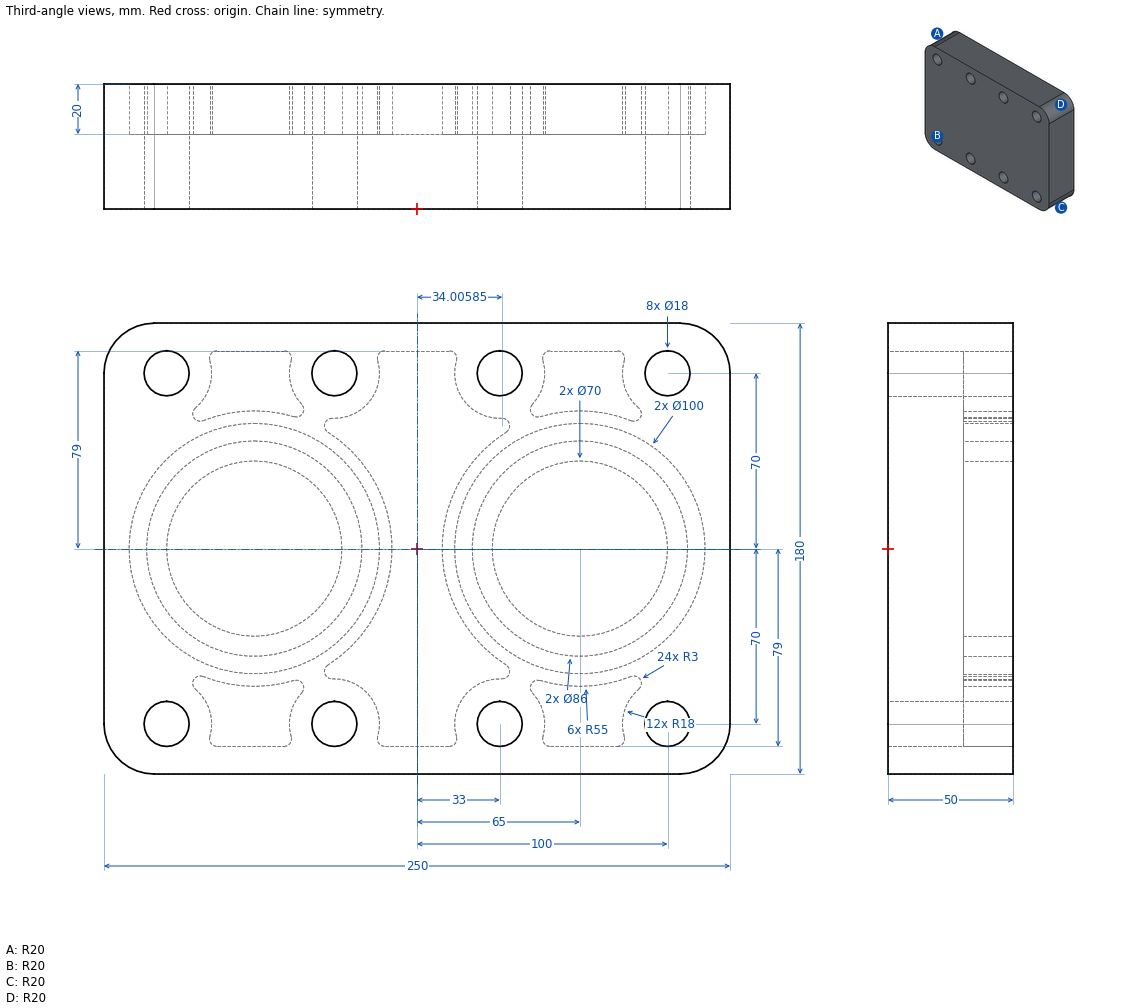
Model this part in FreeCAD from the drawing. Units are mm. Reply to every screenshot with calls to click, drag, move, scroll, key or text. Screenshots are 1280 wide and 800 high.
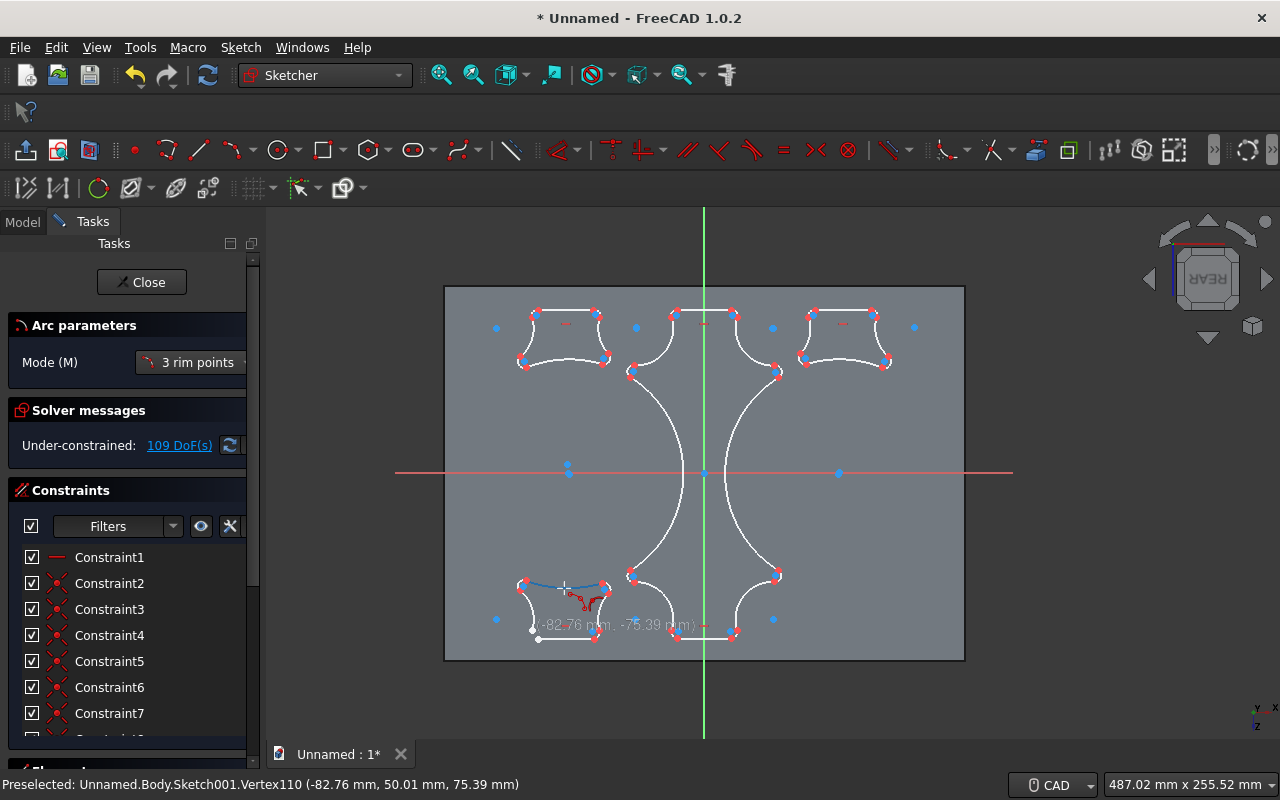
scroll(538, 638, up, 3)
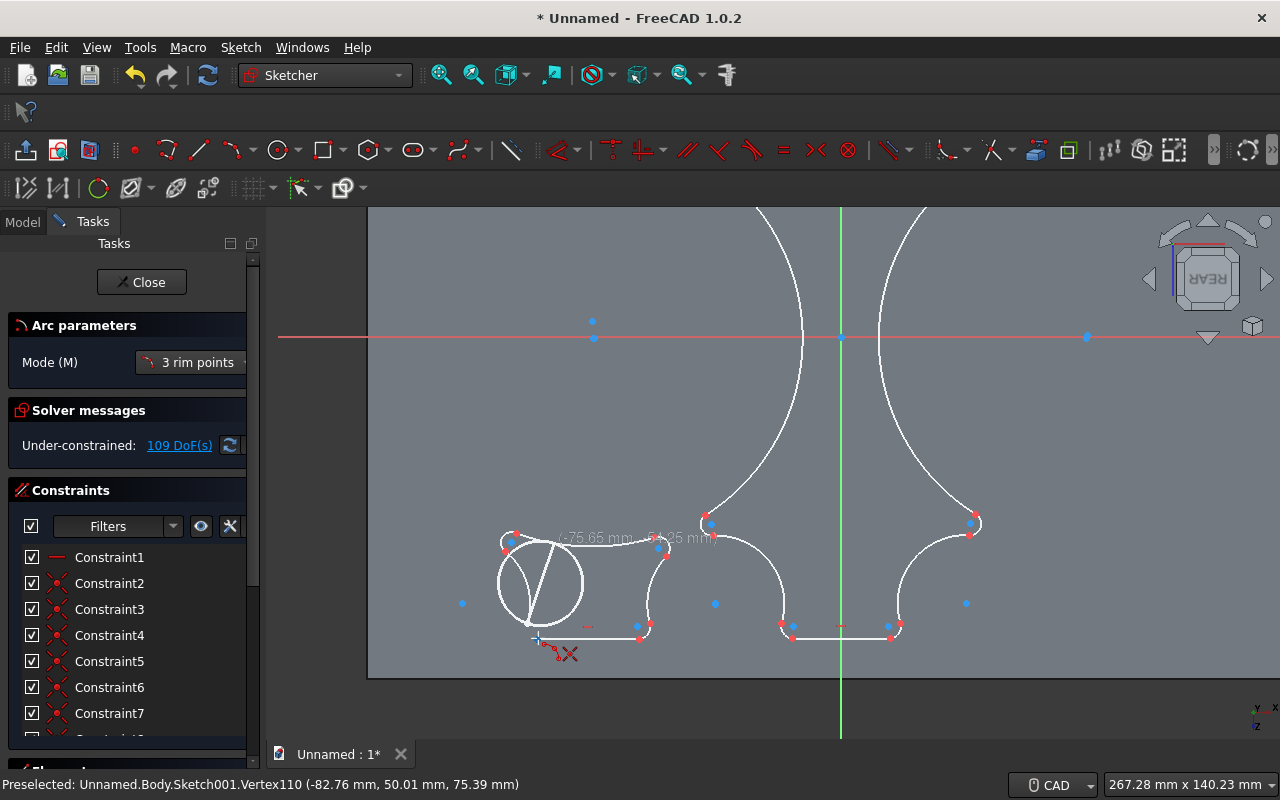
click(538, 639)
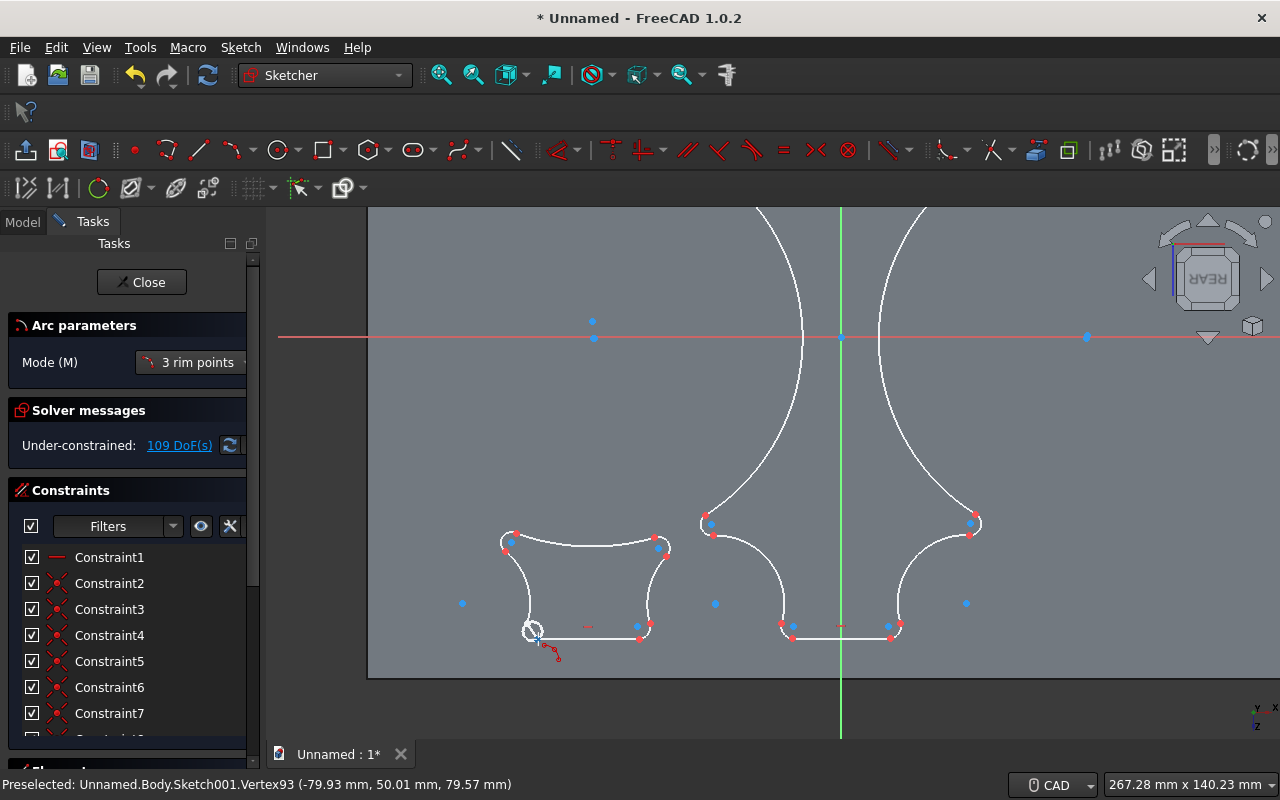
scroll(529, 633, up, 7)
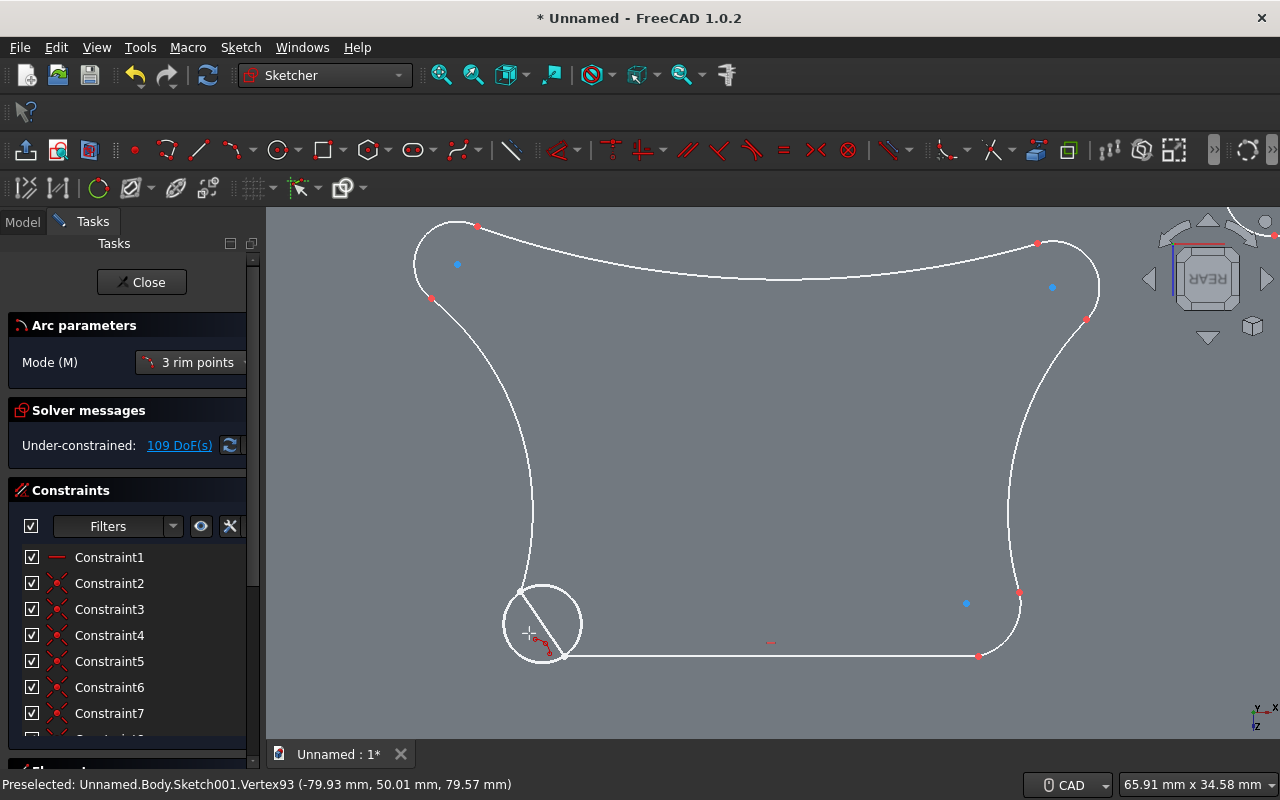
click(528, 629)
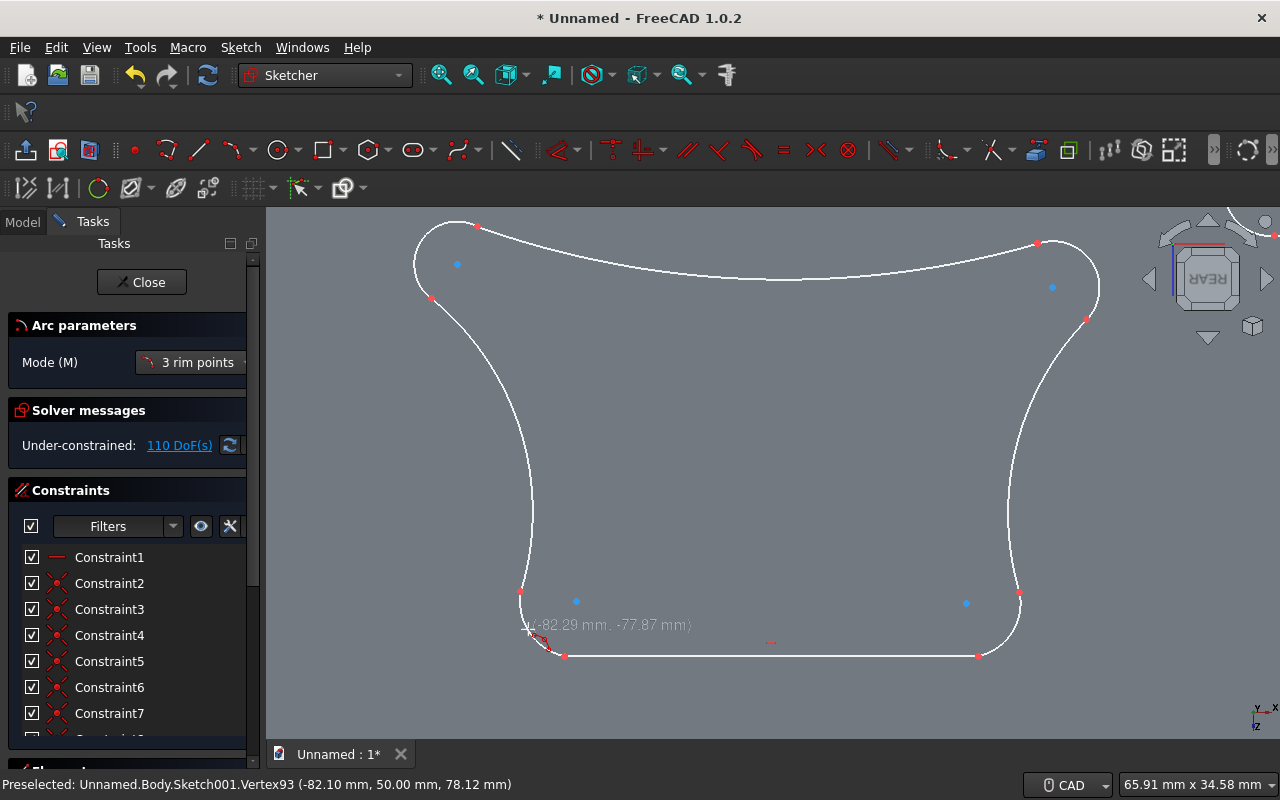
click(200, 150)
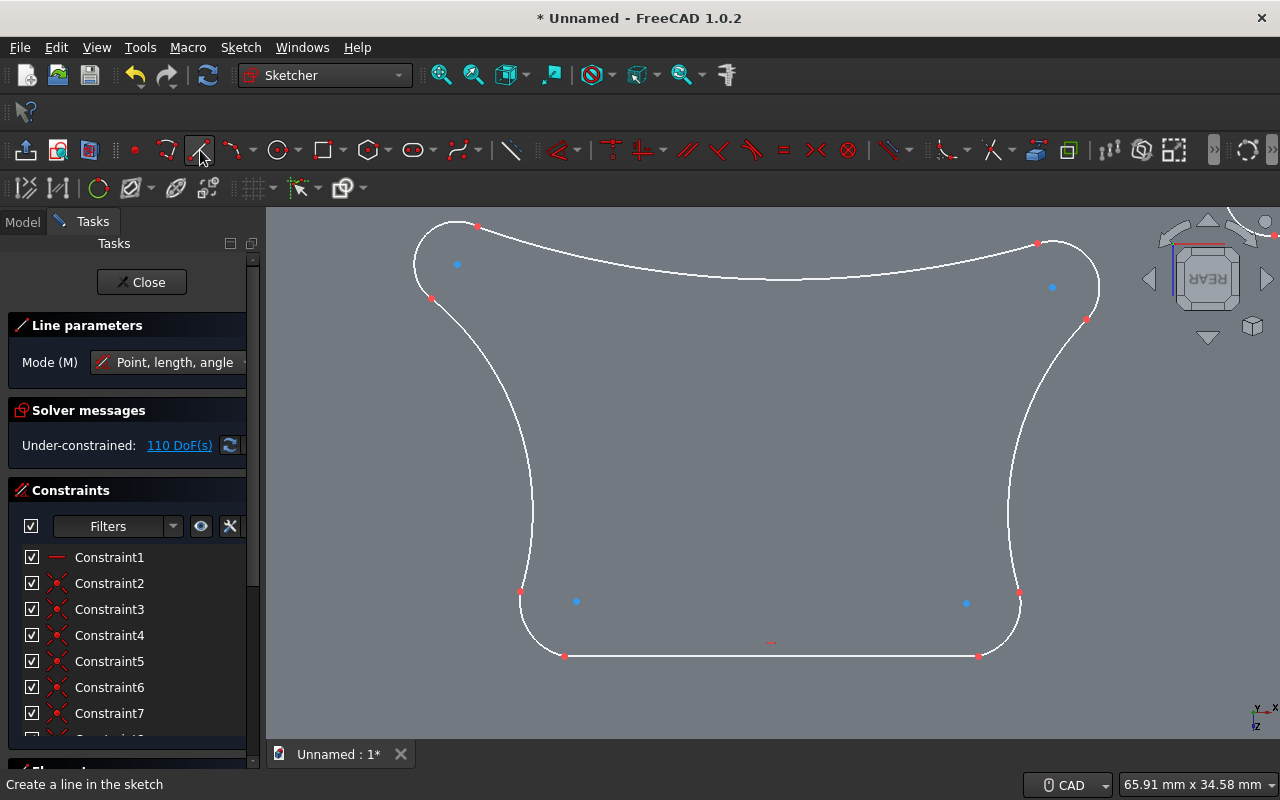
scroll(534, 636, down, 10)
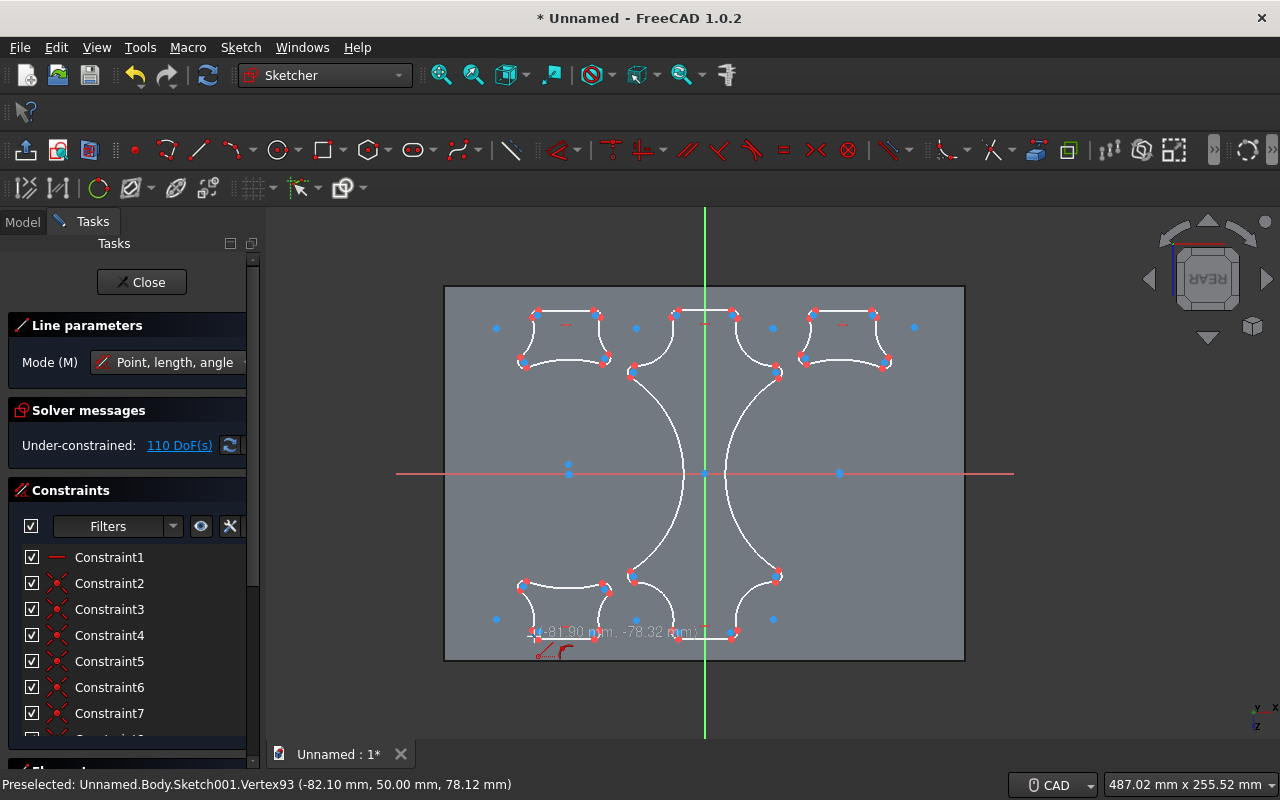
click(815, 638)
click(871, 638)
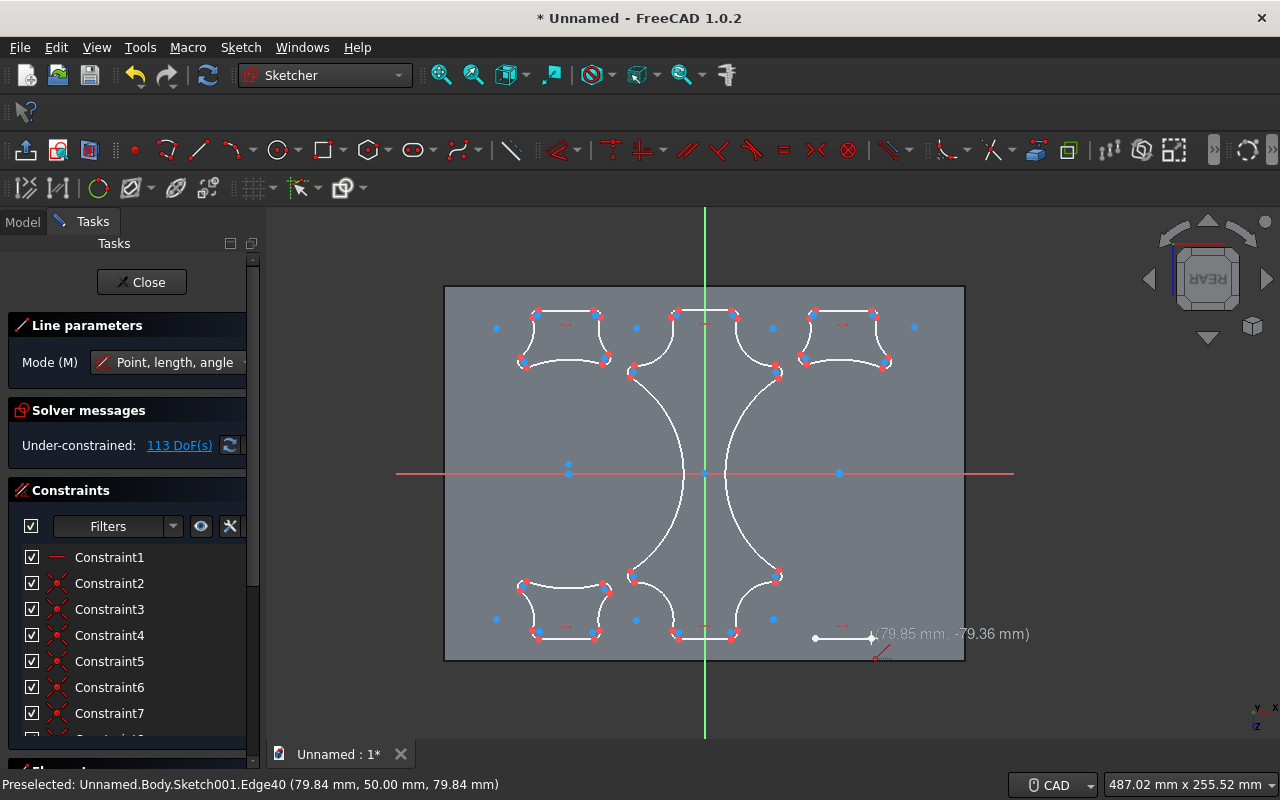
click(232, 150)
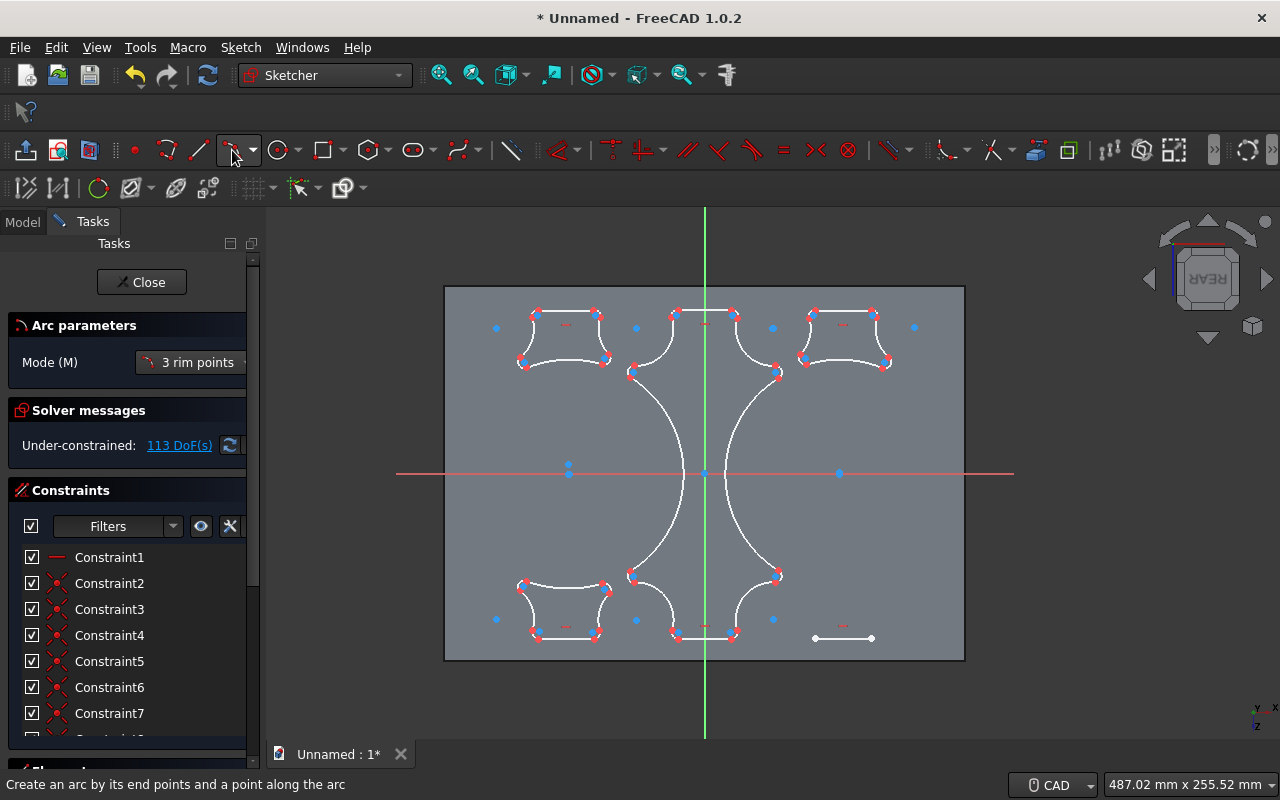
click(871, 639)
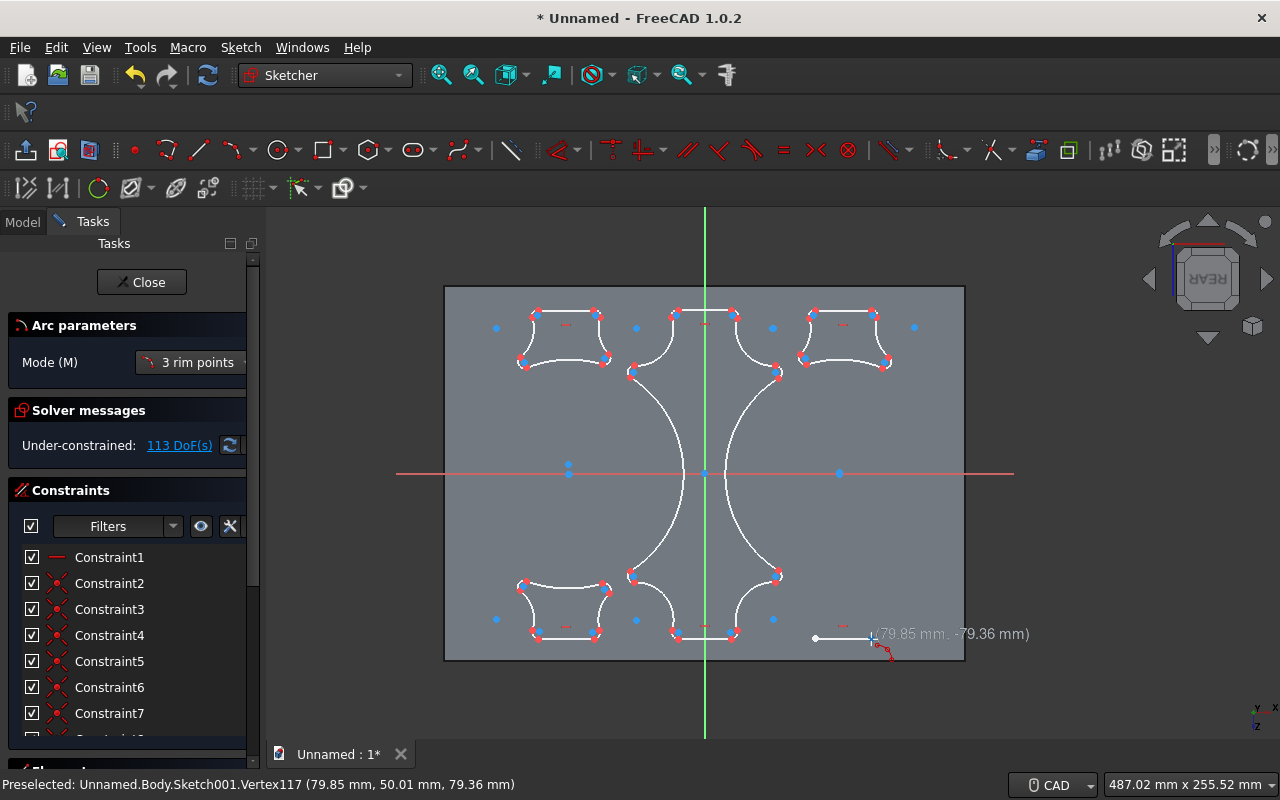
scroll(877, 630, up, 3)